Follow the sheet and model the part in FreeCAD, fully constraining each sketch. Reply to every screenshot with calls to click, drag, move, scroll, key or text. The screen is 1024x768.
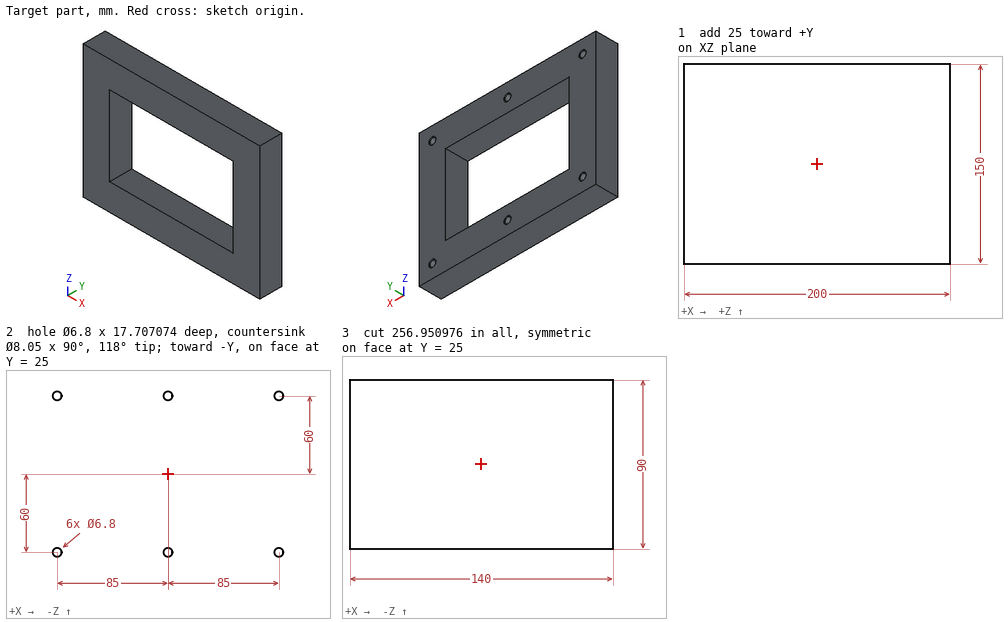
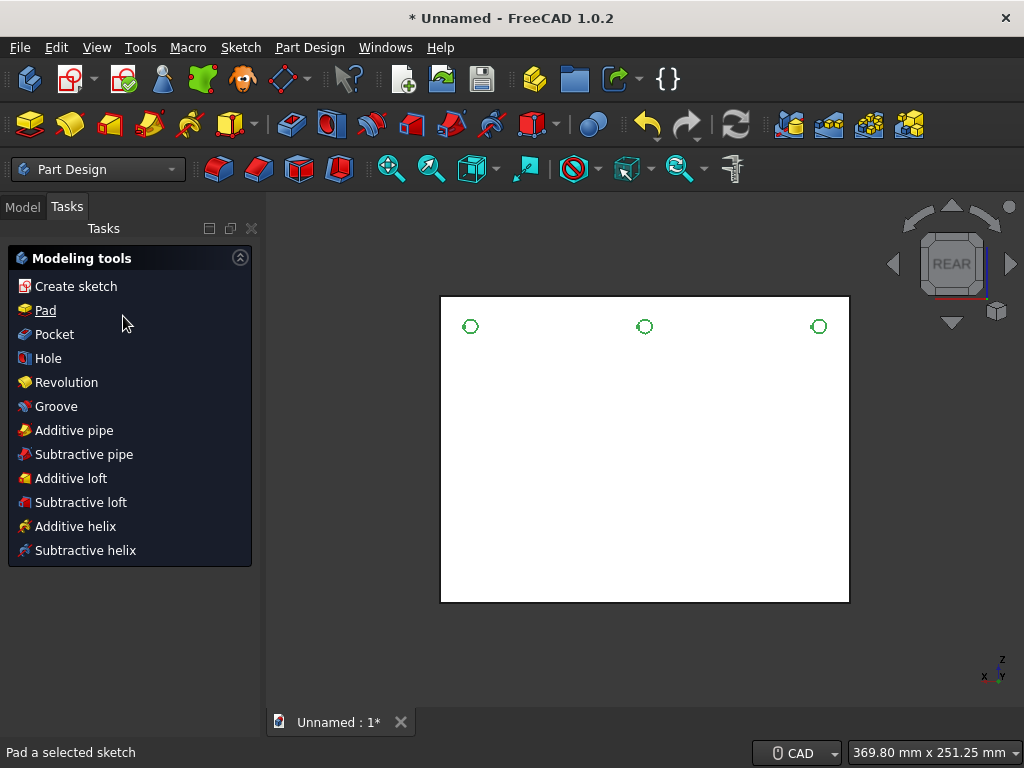
click(332, 124)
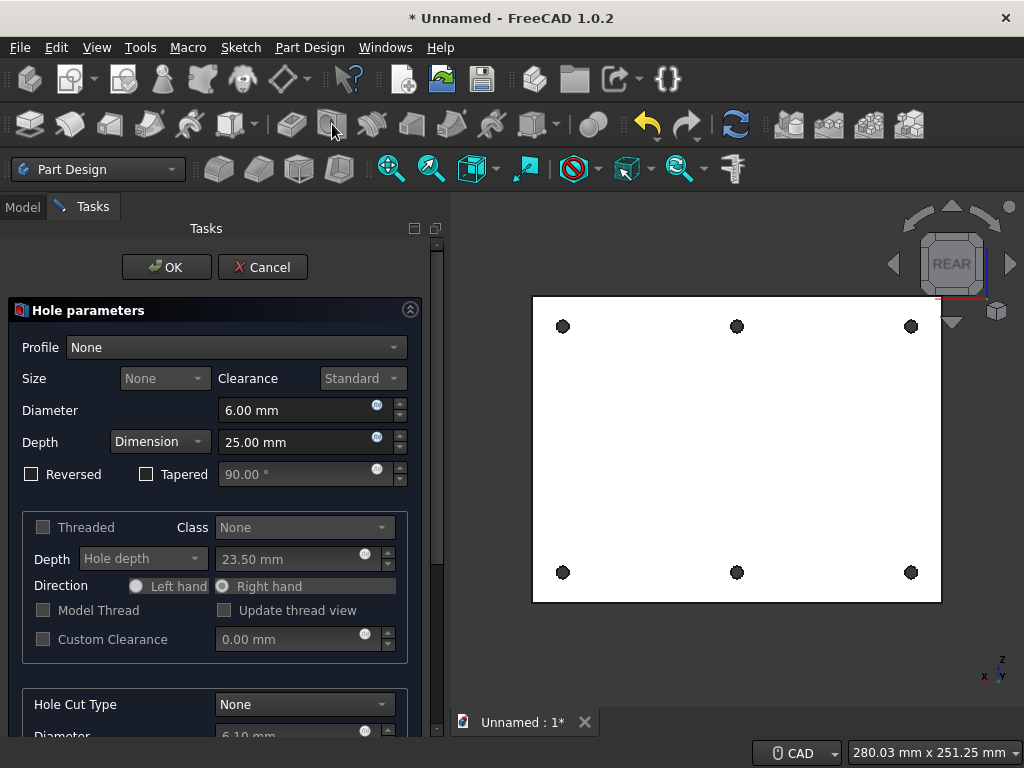
triple_click(305, 410)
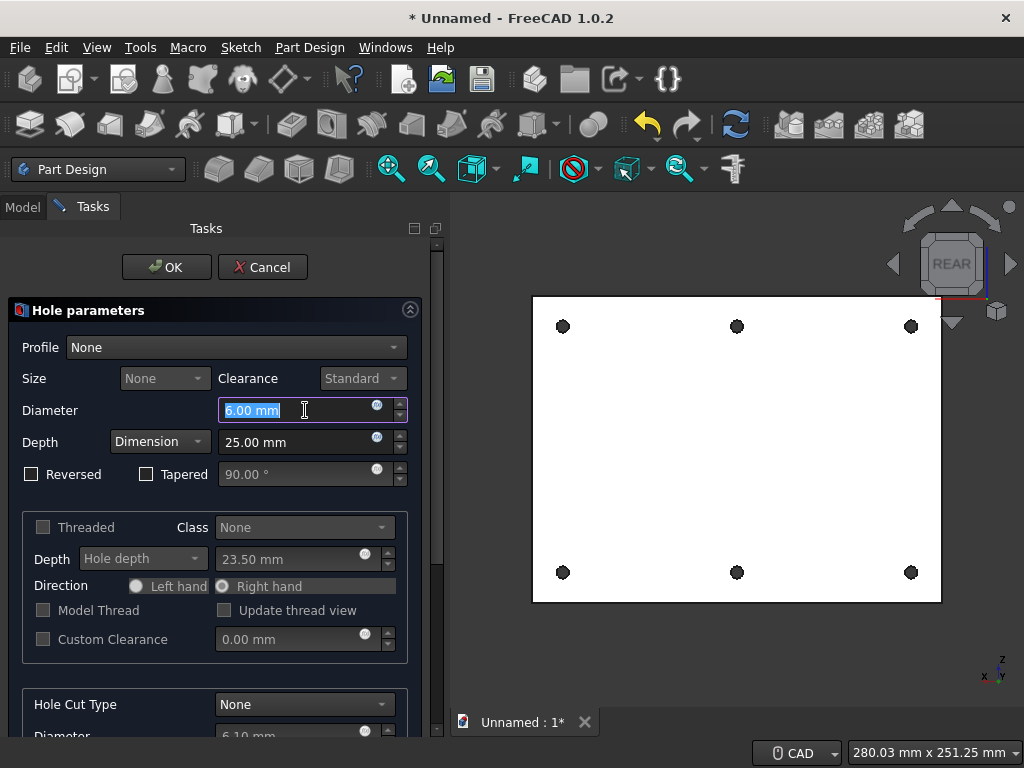
text(6.8)
key(Tab)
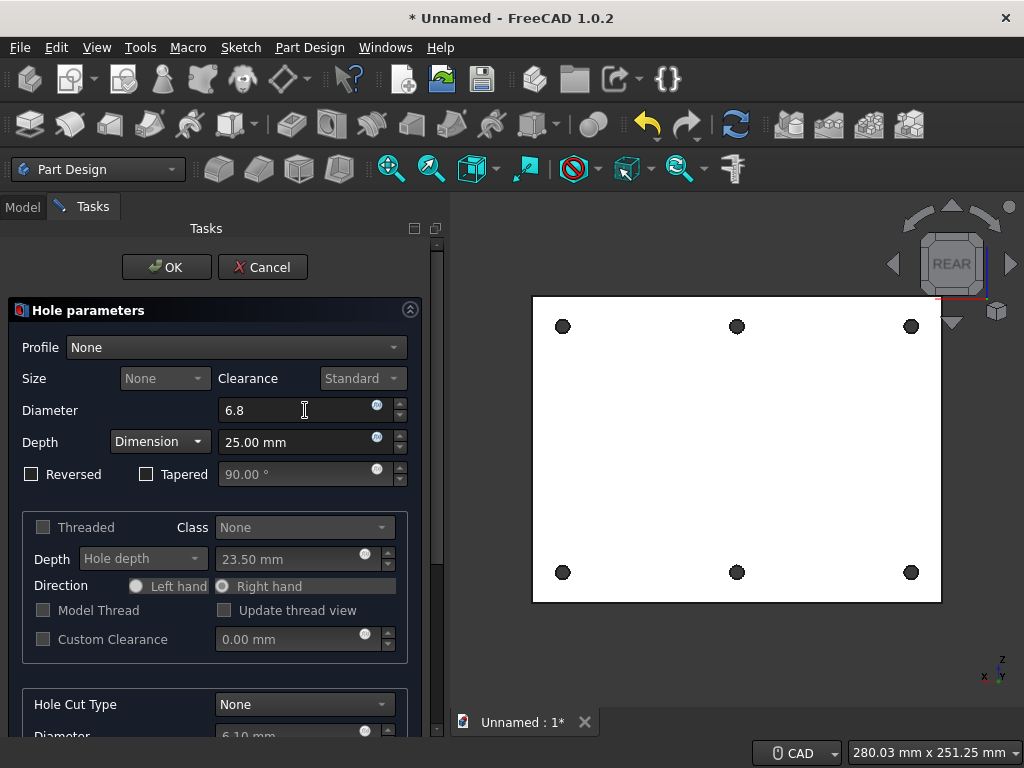
triple_click(305, 442)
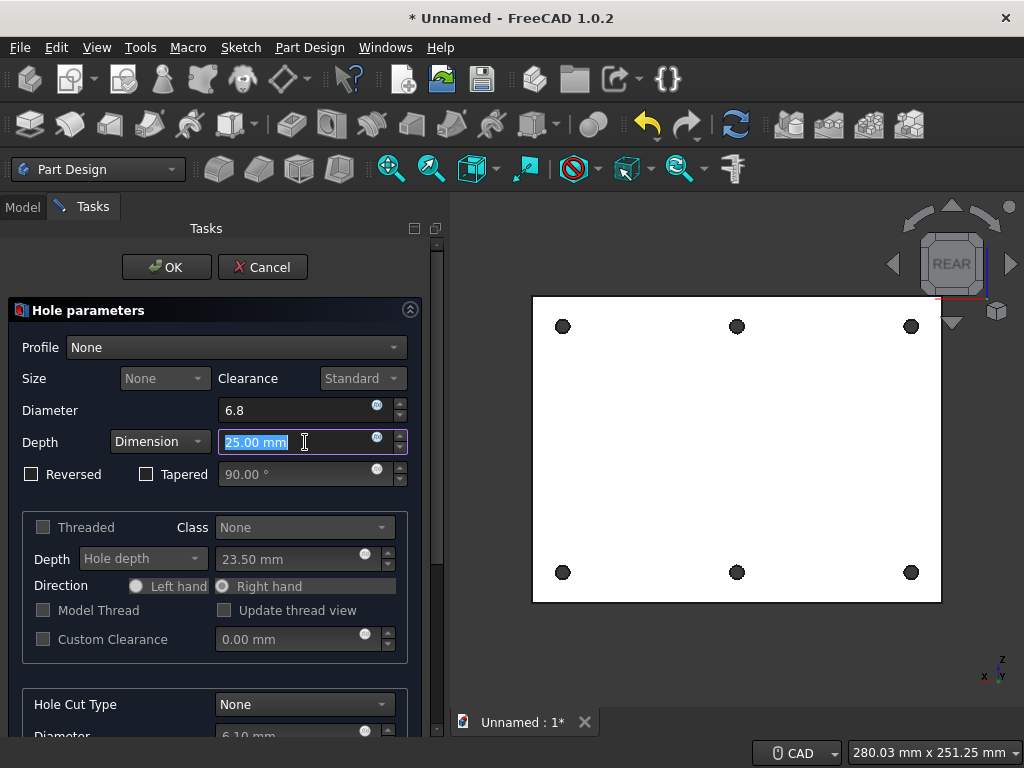
text(17.707074)
key(Tab)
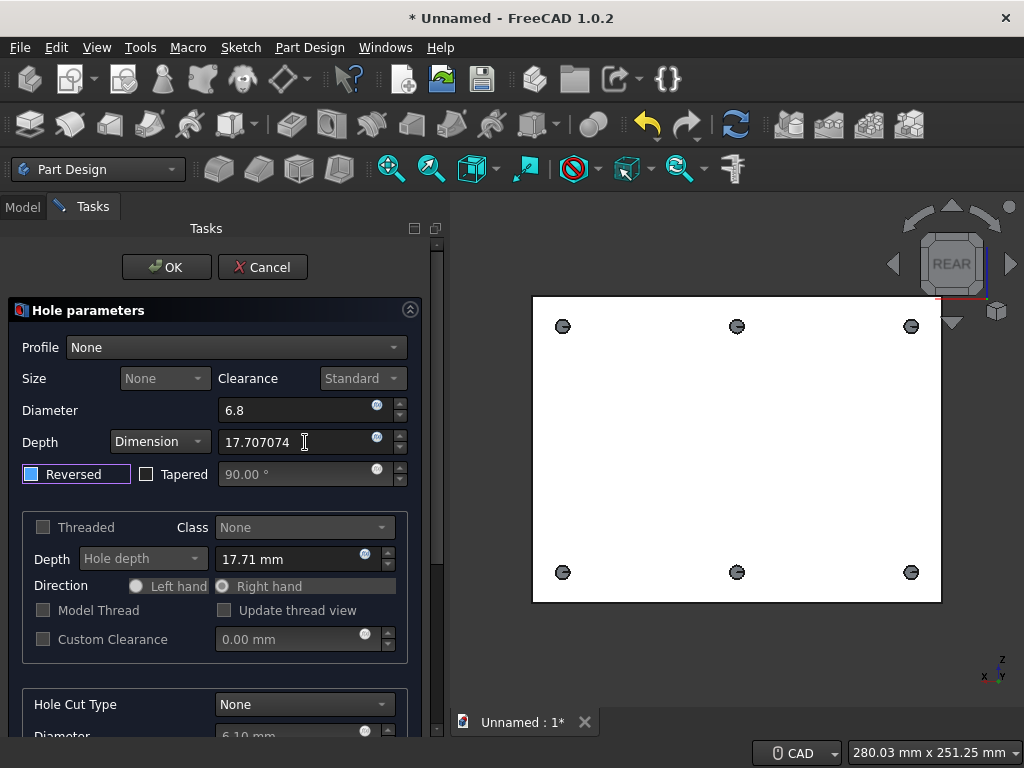
click(306, 704)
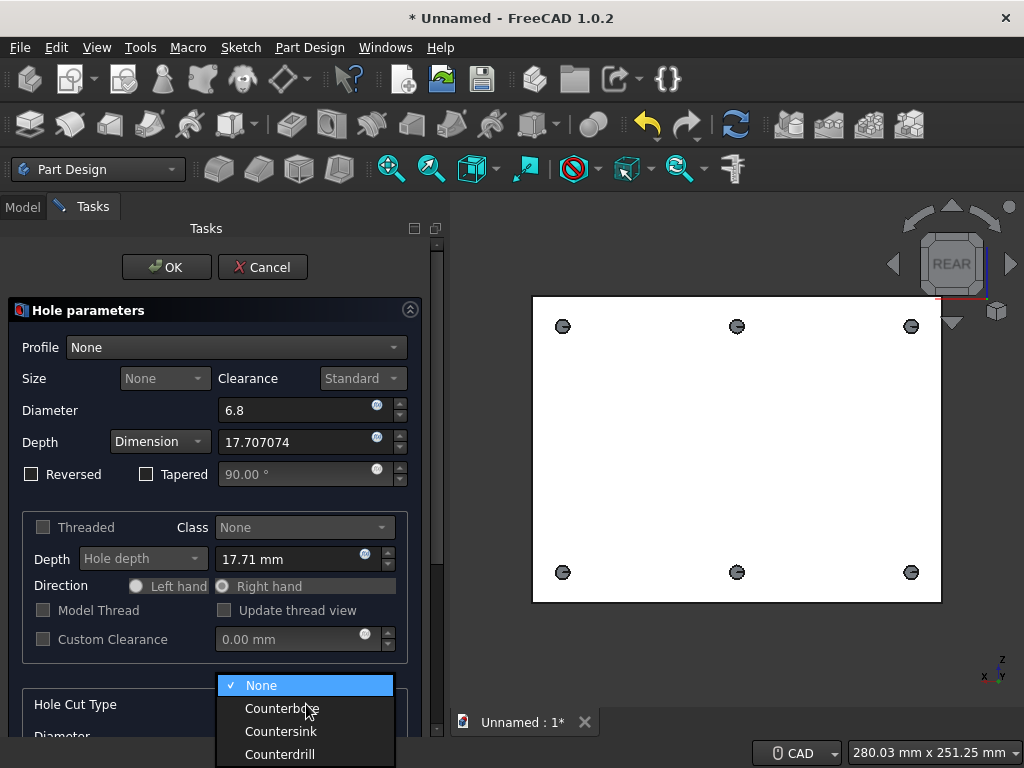
click(304, 732)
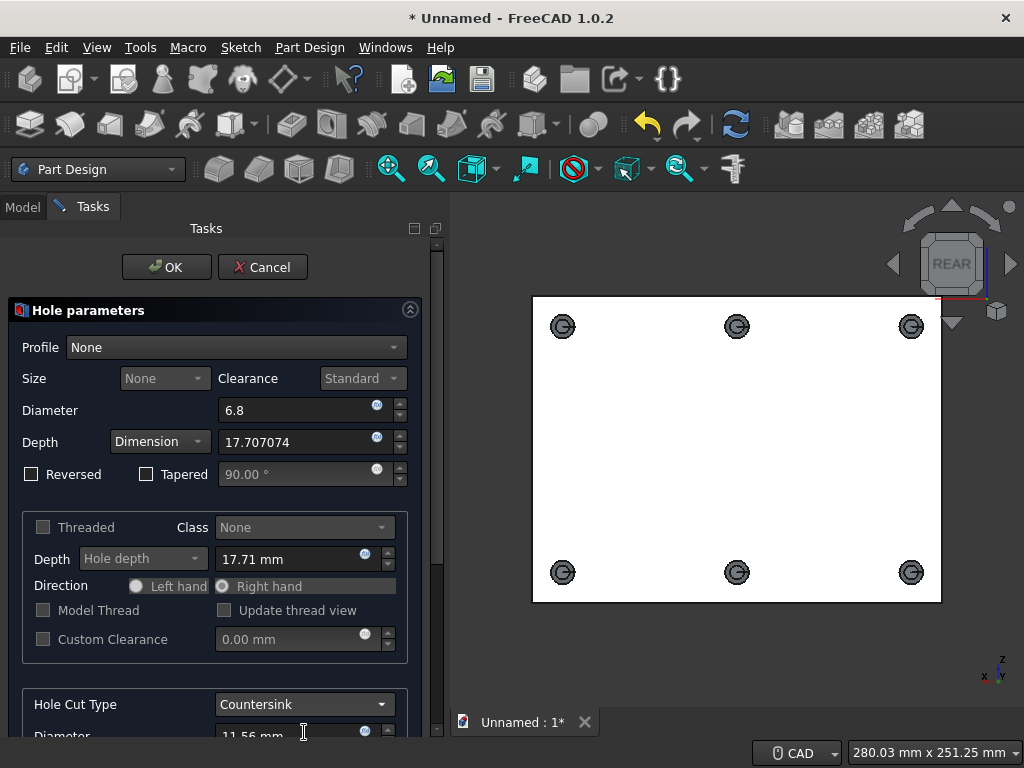
scroll(437, 487, down, 2)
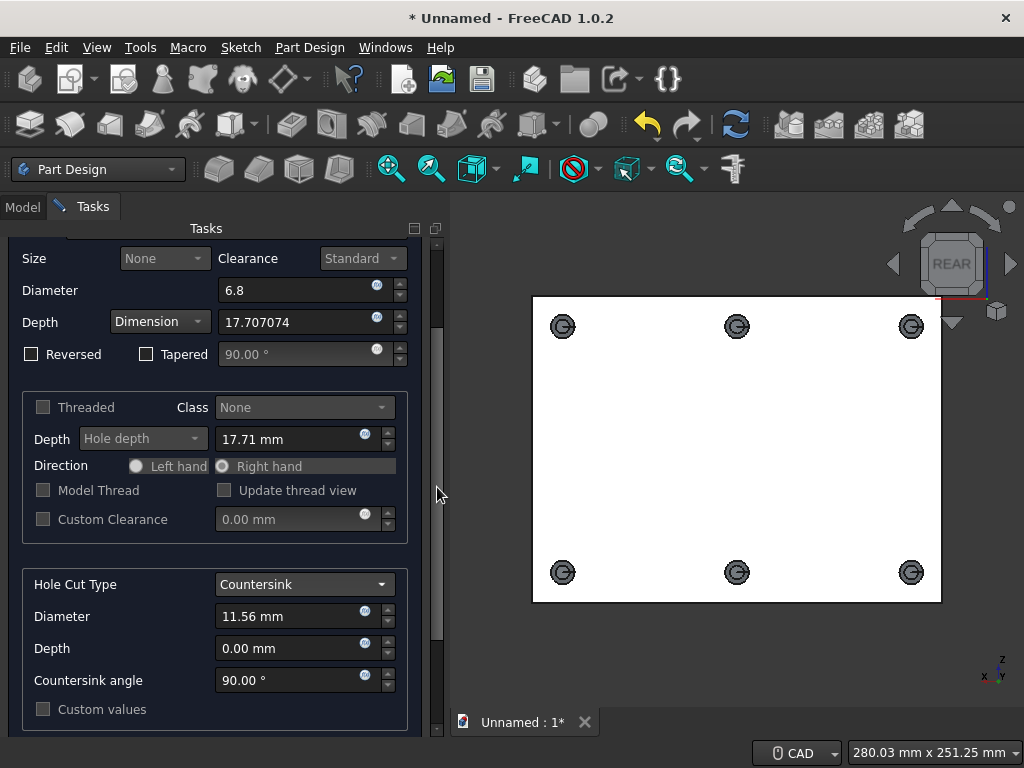
triple_click(298, 616)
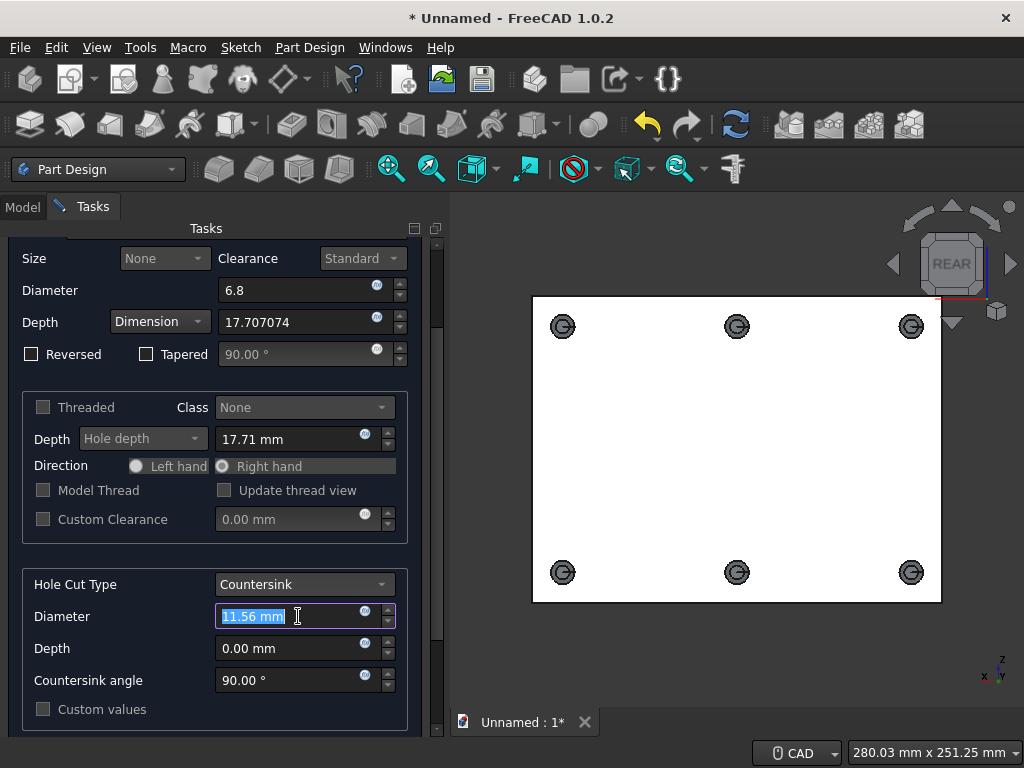
text(8.05)
key(Tab)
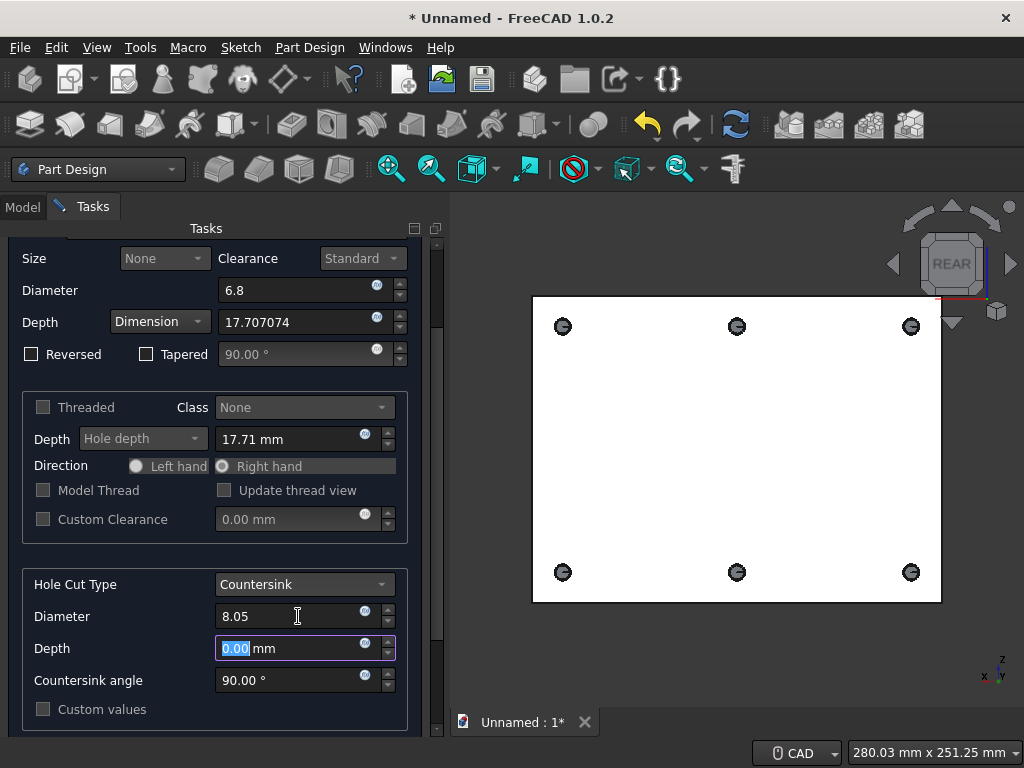
scroll(437, 487, up, 3)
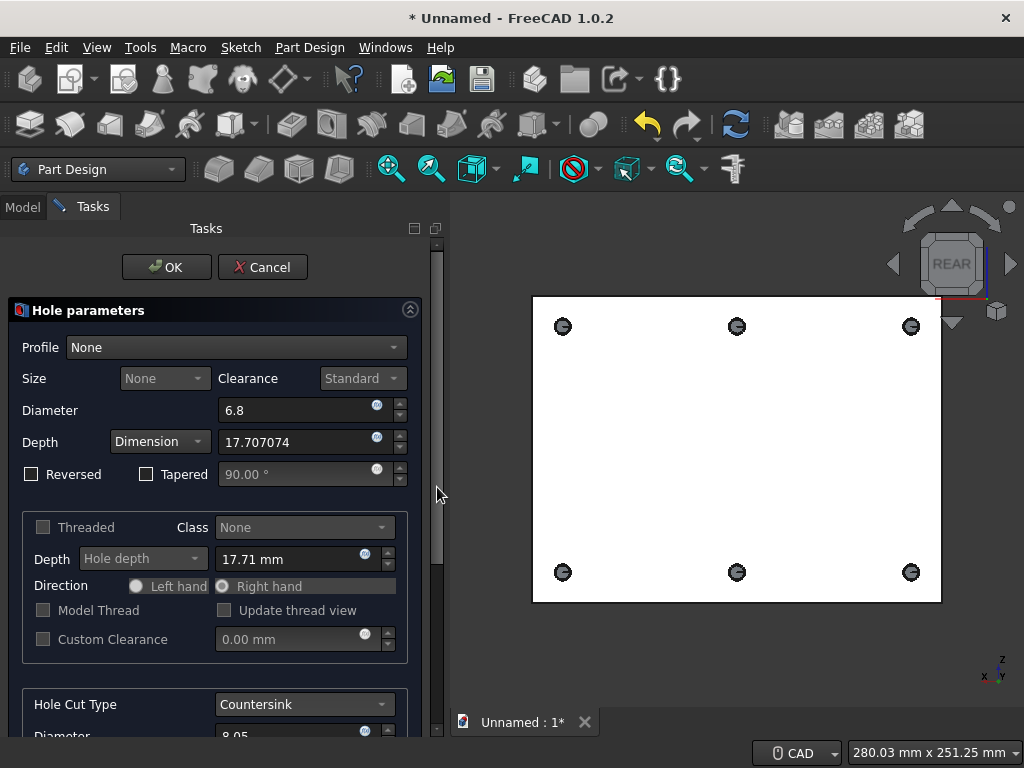
click(167, 267)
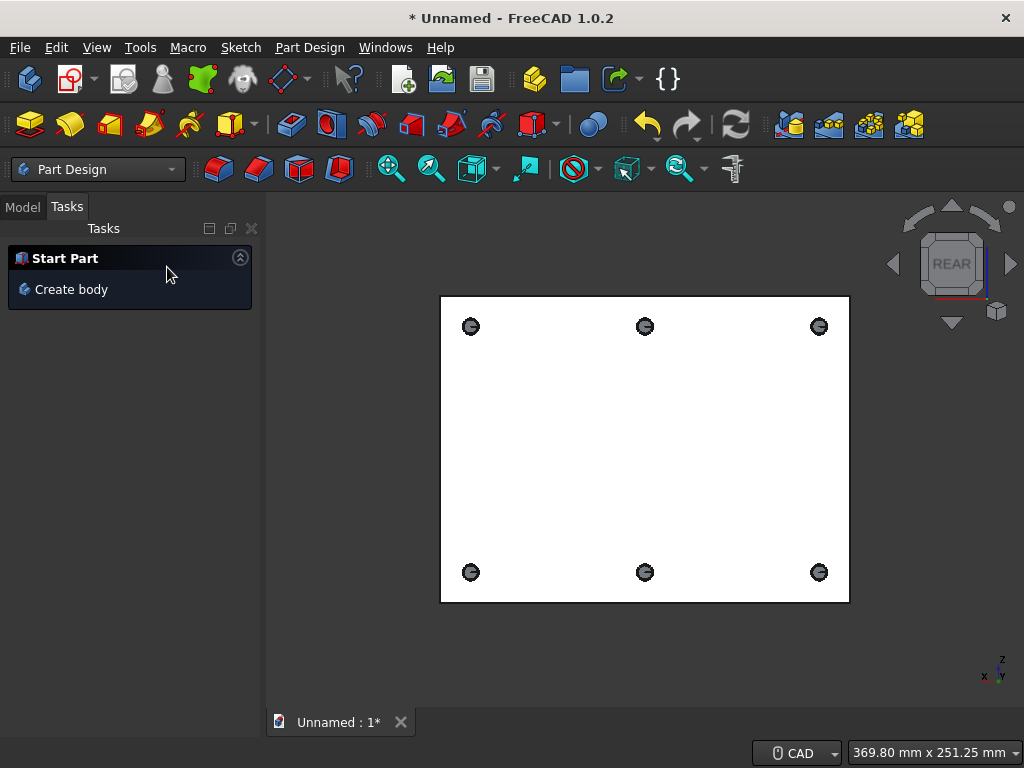
click(586, 448)